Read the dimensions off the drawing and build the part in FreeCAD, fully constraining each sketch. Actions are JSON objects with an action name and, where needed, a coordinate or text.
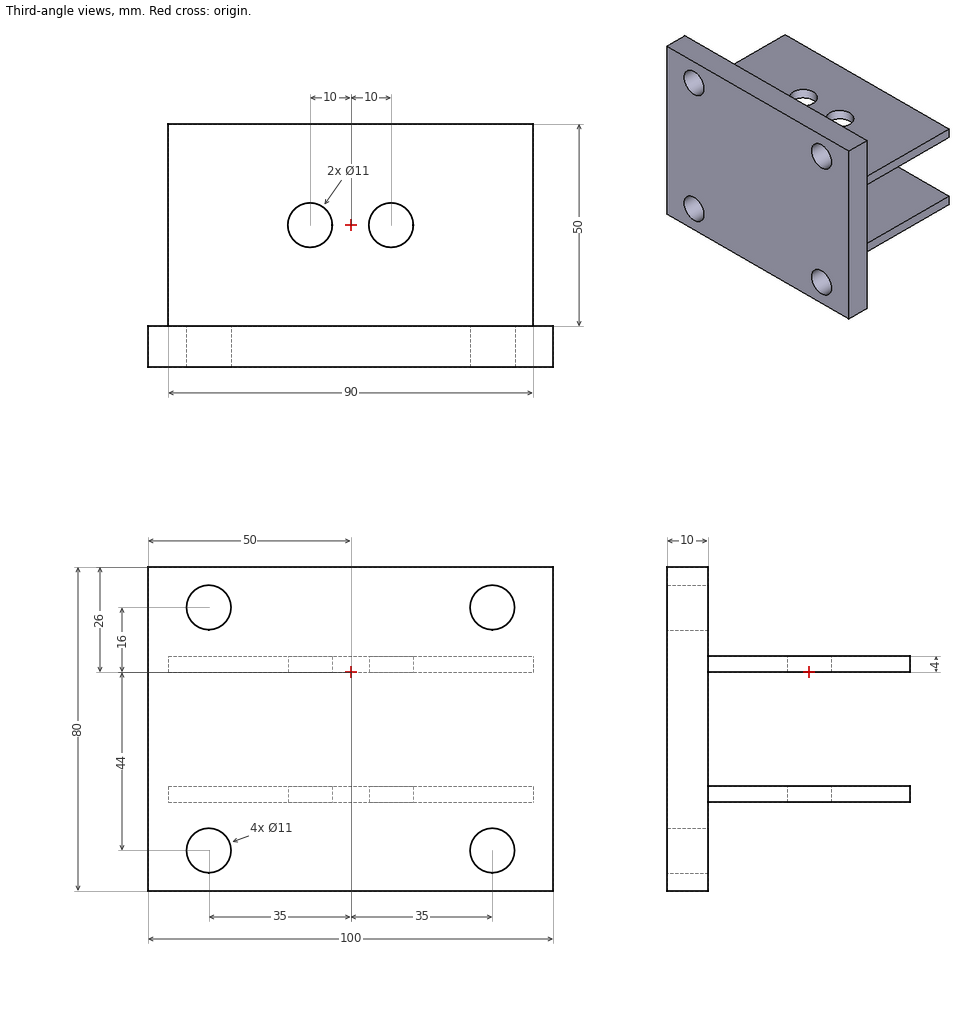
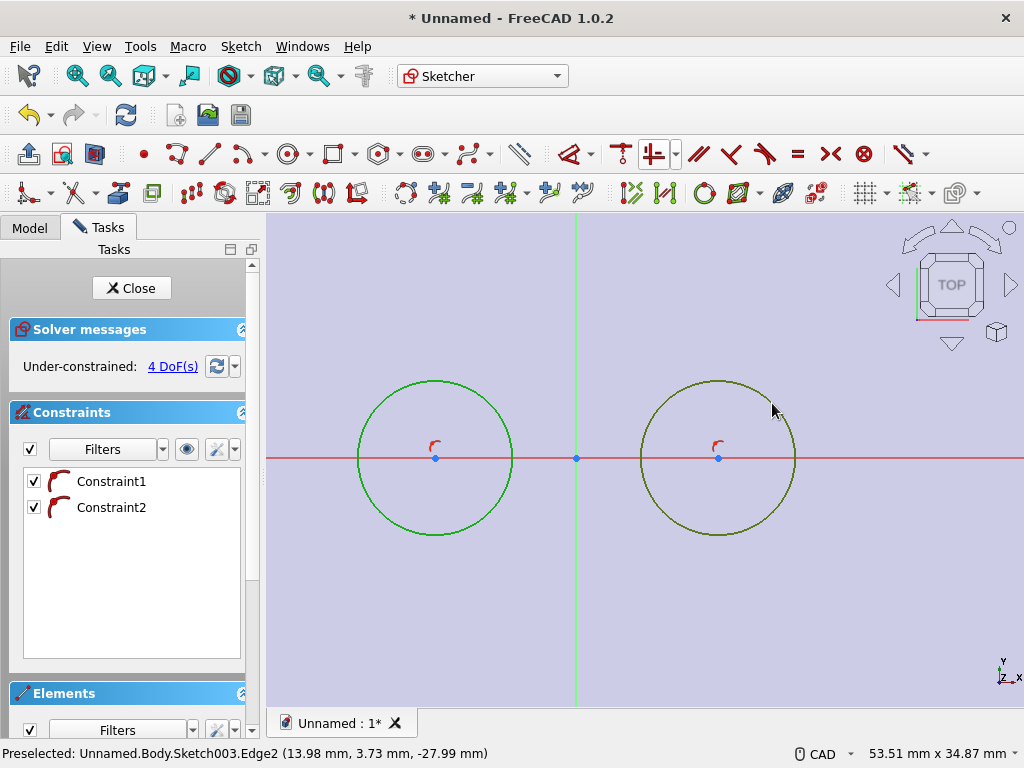
{"action": "key", "text": "e"}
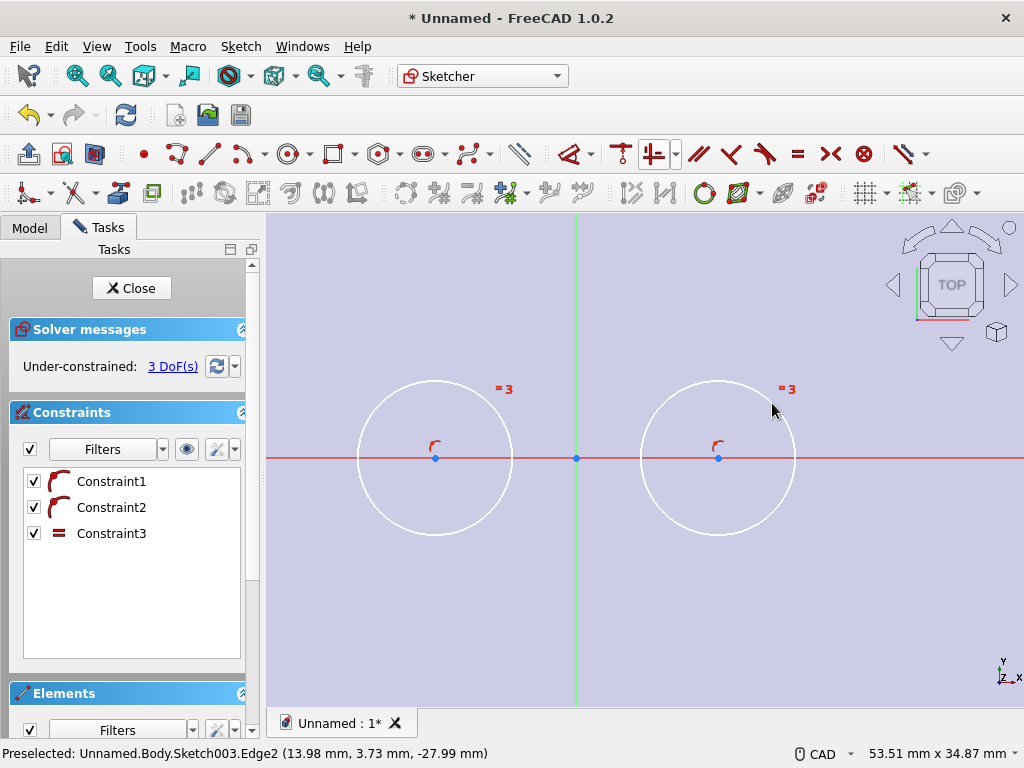
{"action": "key", "text": "d"}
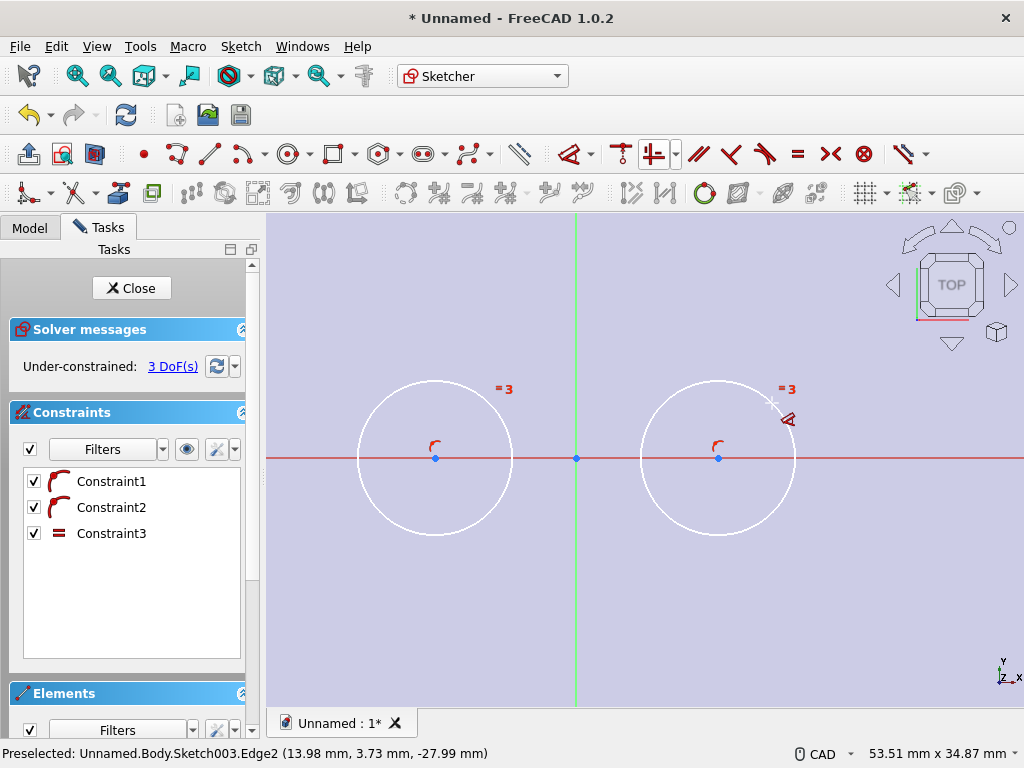
{"action": "left_click", "coordinate": [489, 403]}
{"action": "left_click", "coordinate": [511, 380]}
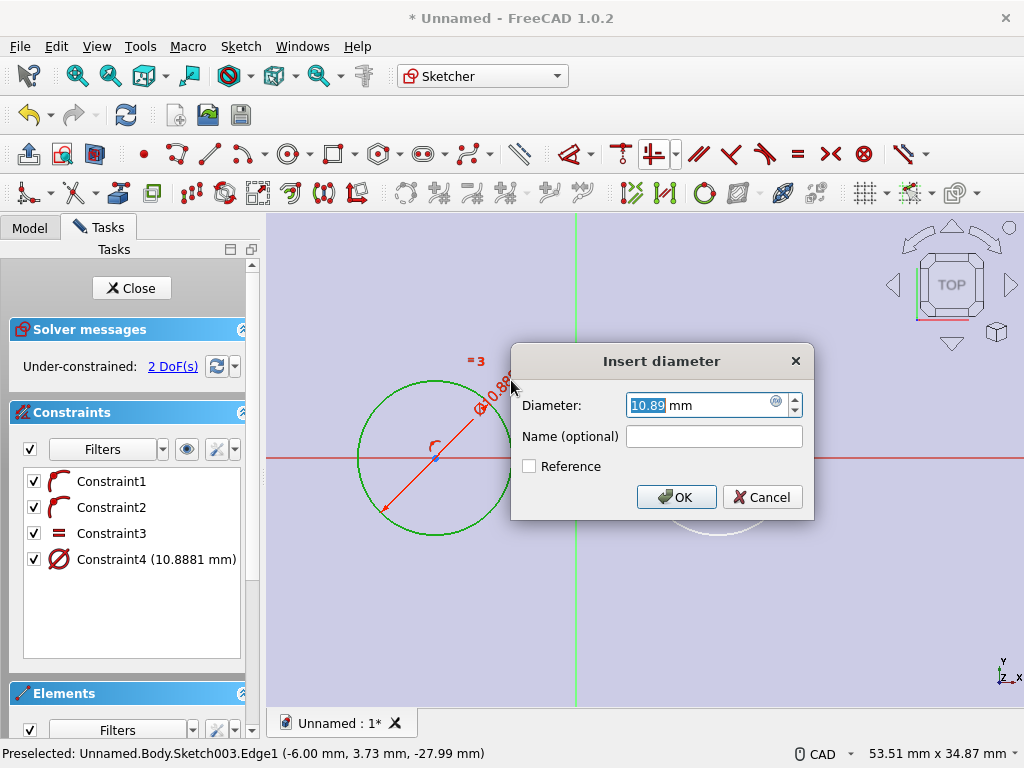
{"action": "type", "text": "11"}
{"action": "key", "text": "Return"}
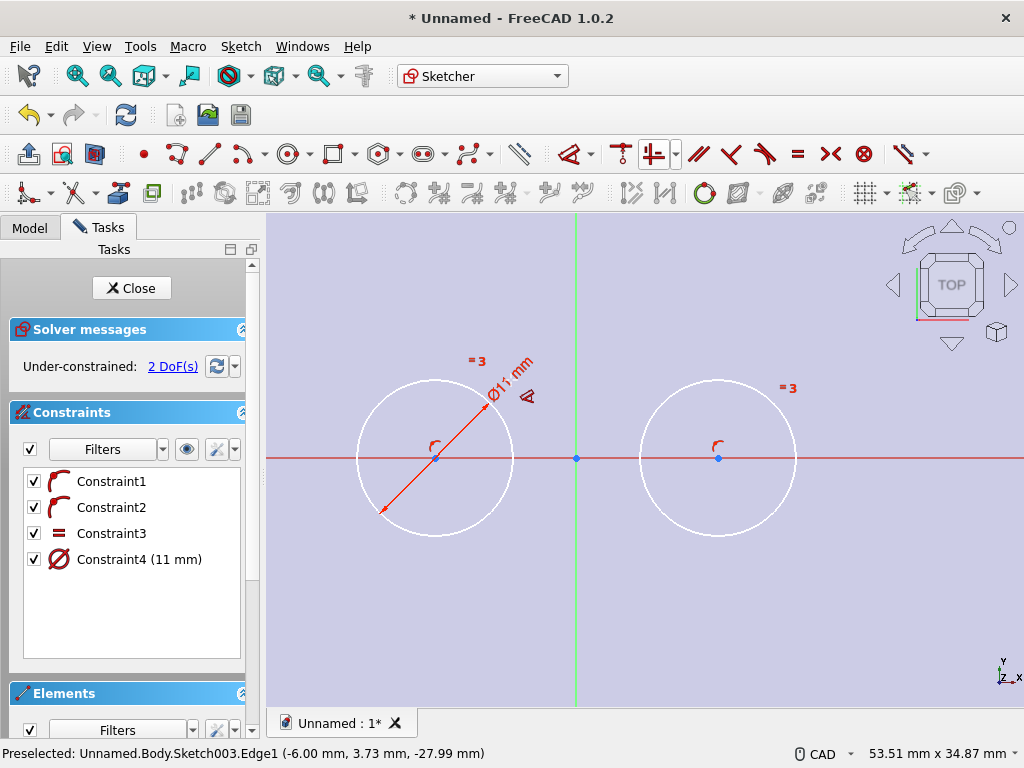
{"action": "left_click", "coordinate": [435, 458]}
{"action": "left_click", "coordinate": [473, 492]}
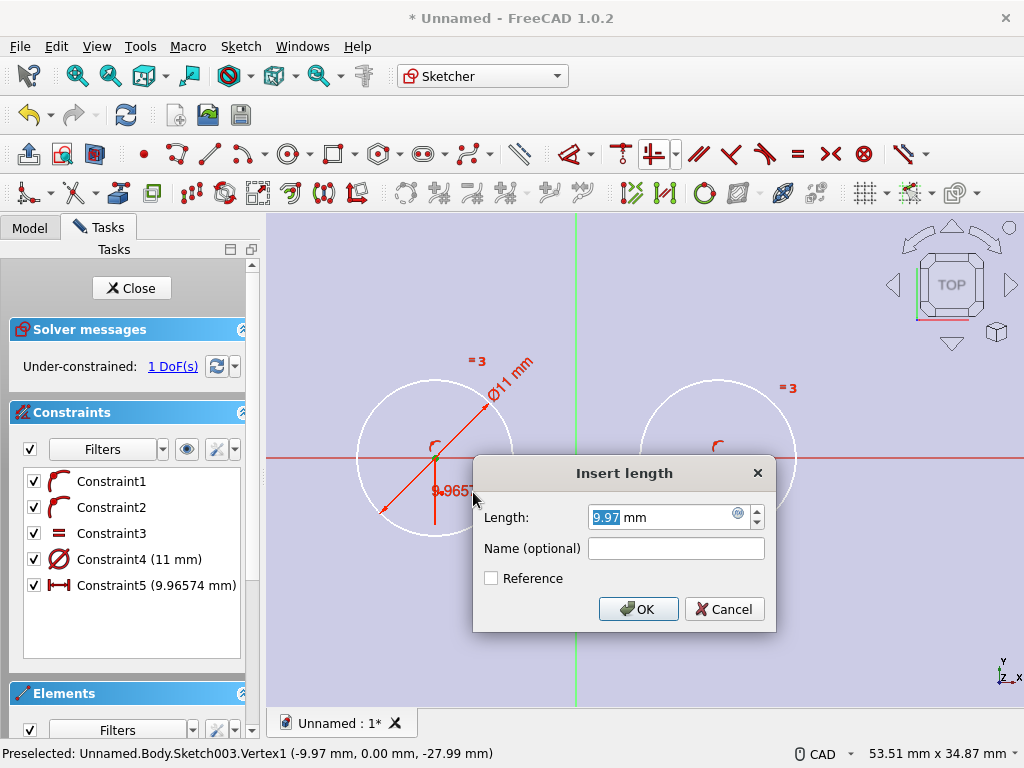
{"action": "type", "text": "10"}
{"action": "key", "text": "Return"}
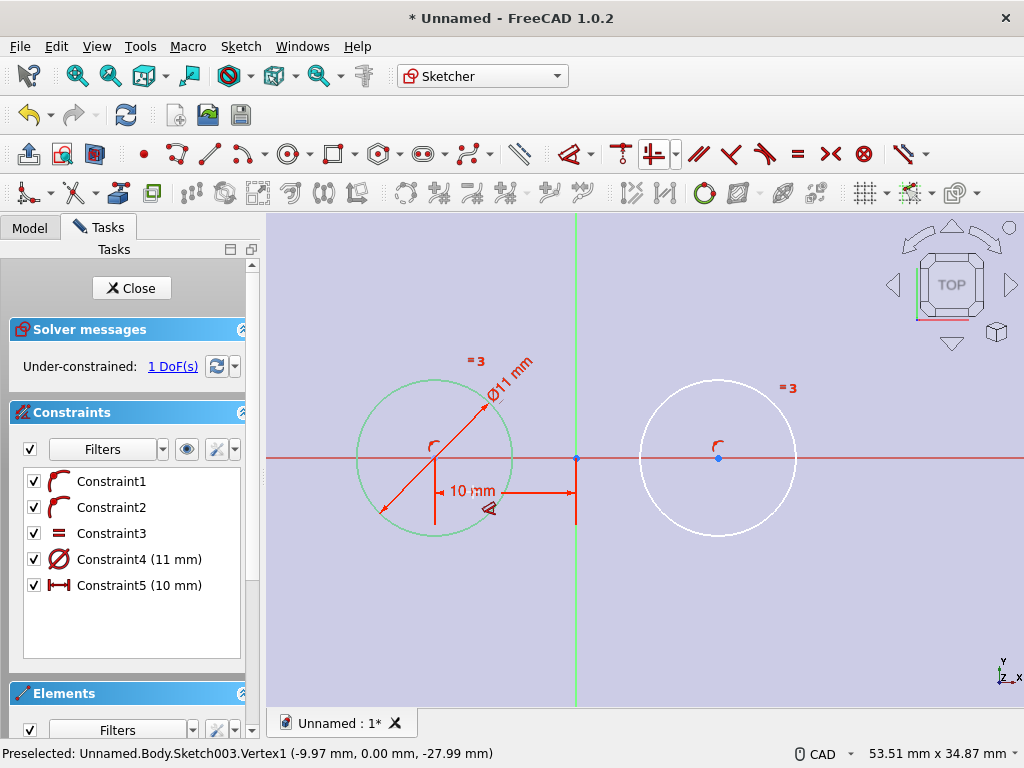
{"action": "left_click", "coordinate": [718, 458]}
{"action": "left_click", "coordinate": [614, 492]}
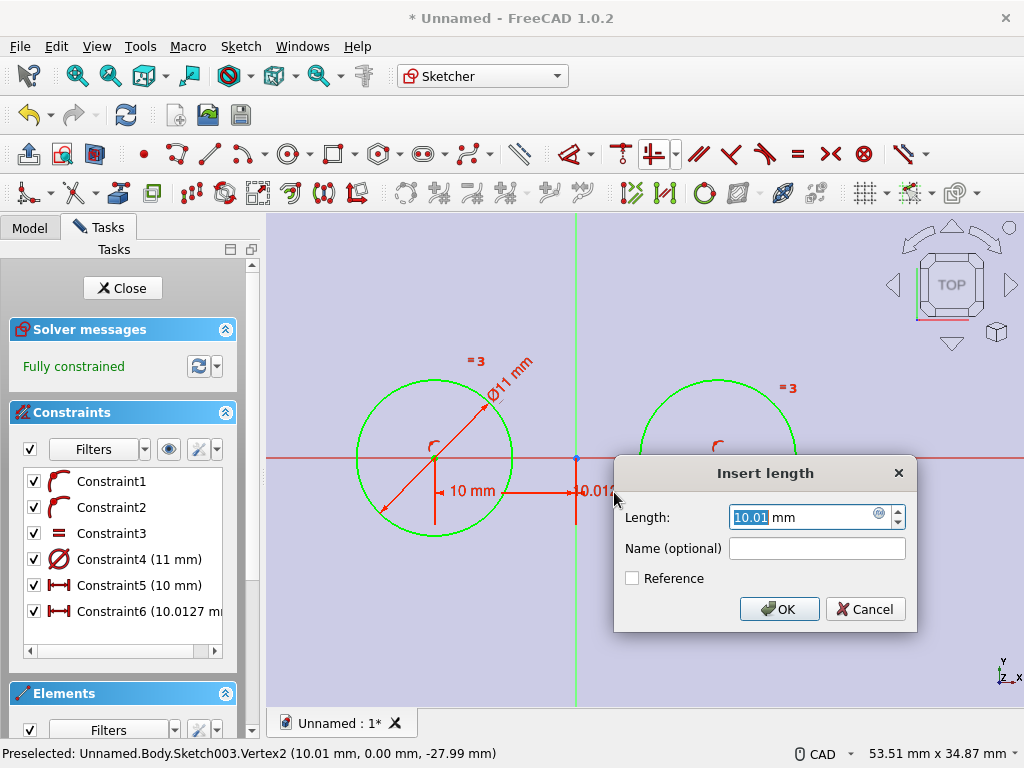
{"action": "type", "text": "10"}
{"action": "key", "text": "Return"}
{"action": "key", "text": "Escape"}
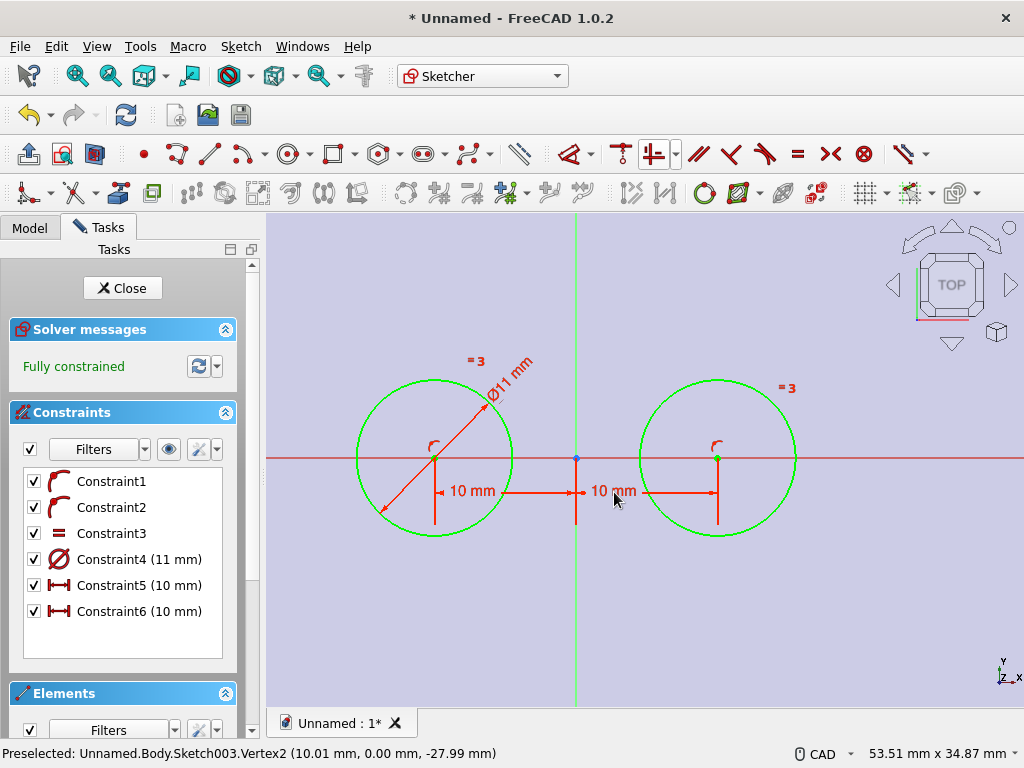
{"action": "left_click", "coordinate": [123, 288]}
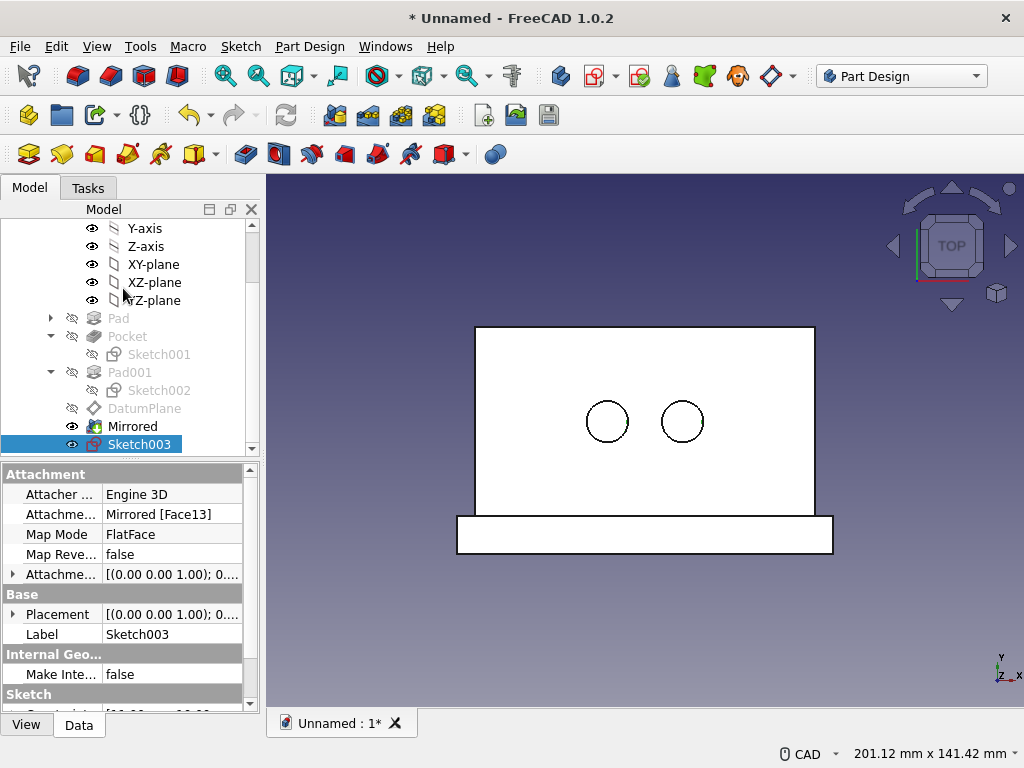
{"action": "left_click", "coordinate": [246, 154]}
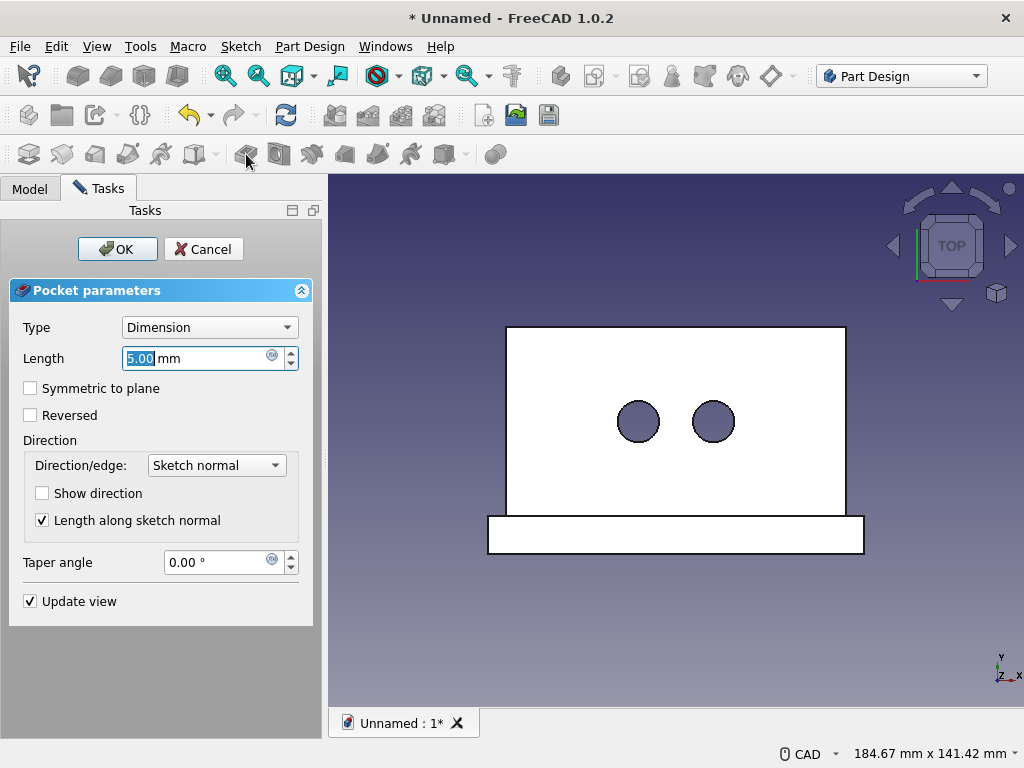
{"action": "left_click", "coordinate": [210, 328]}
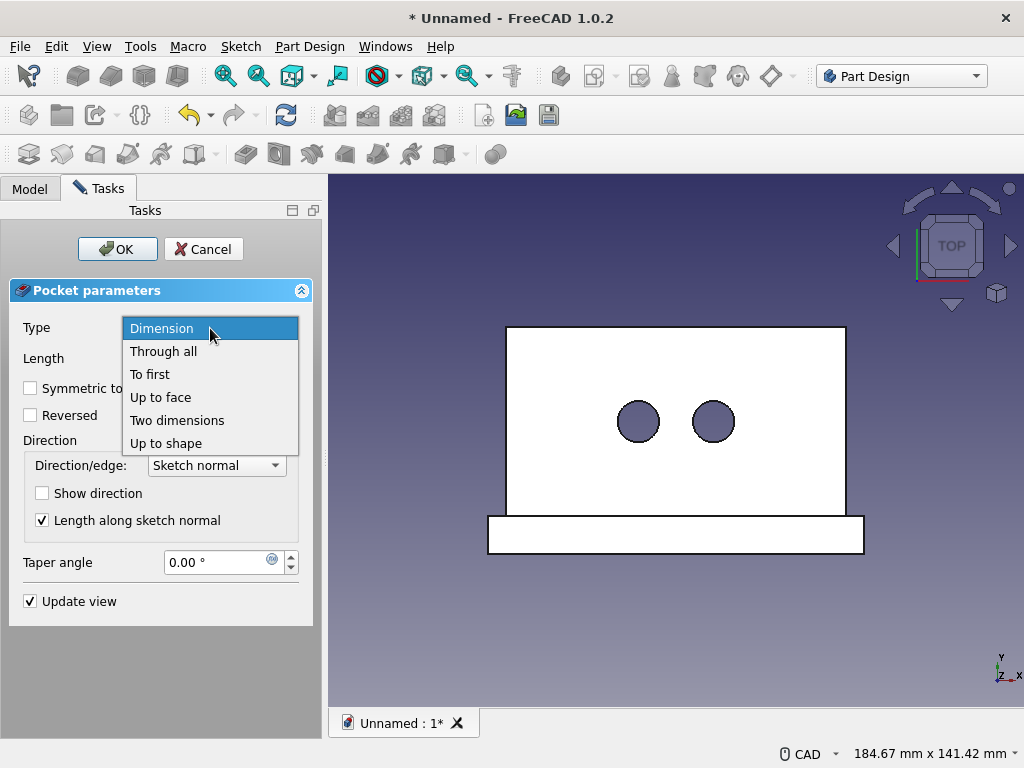
{"action": "left_click", "coordinate": [208, 352]}